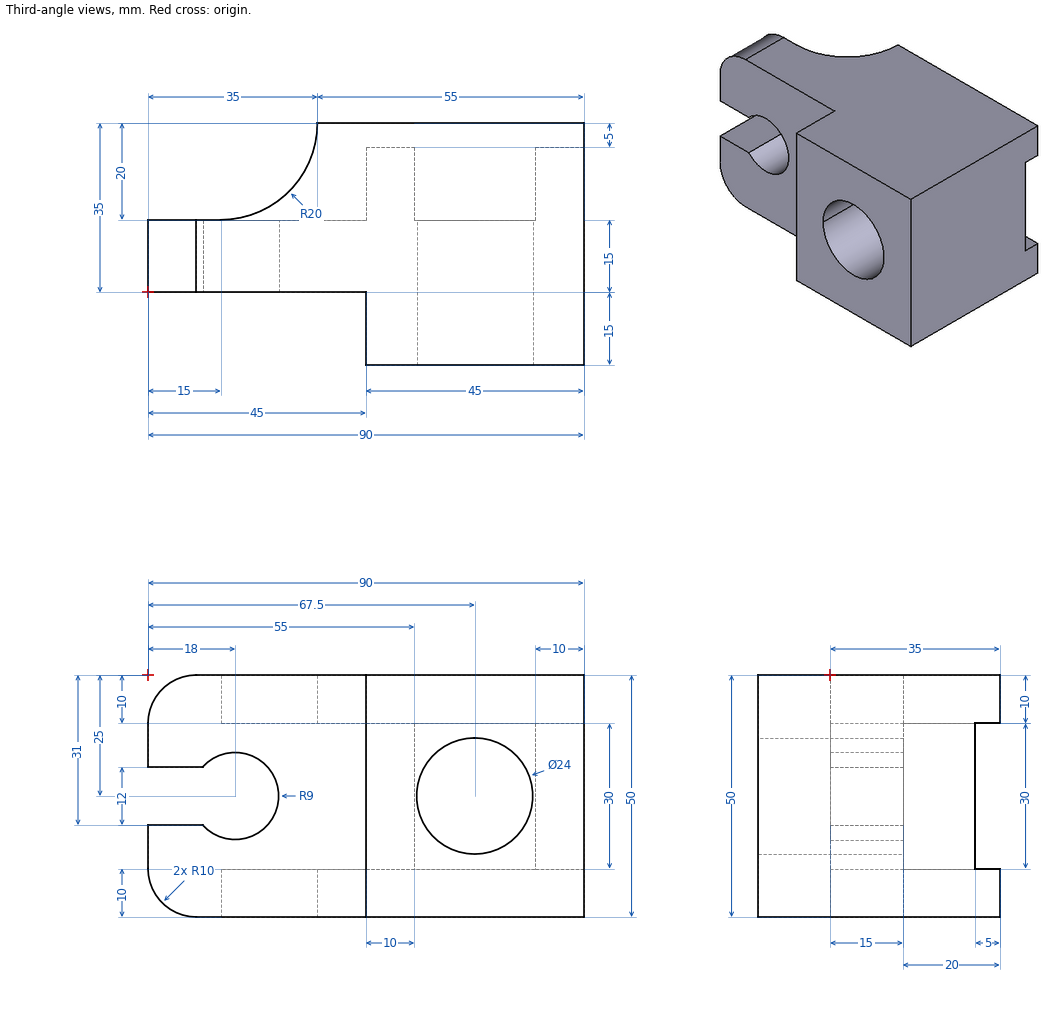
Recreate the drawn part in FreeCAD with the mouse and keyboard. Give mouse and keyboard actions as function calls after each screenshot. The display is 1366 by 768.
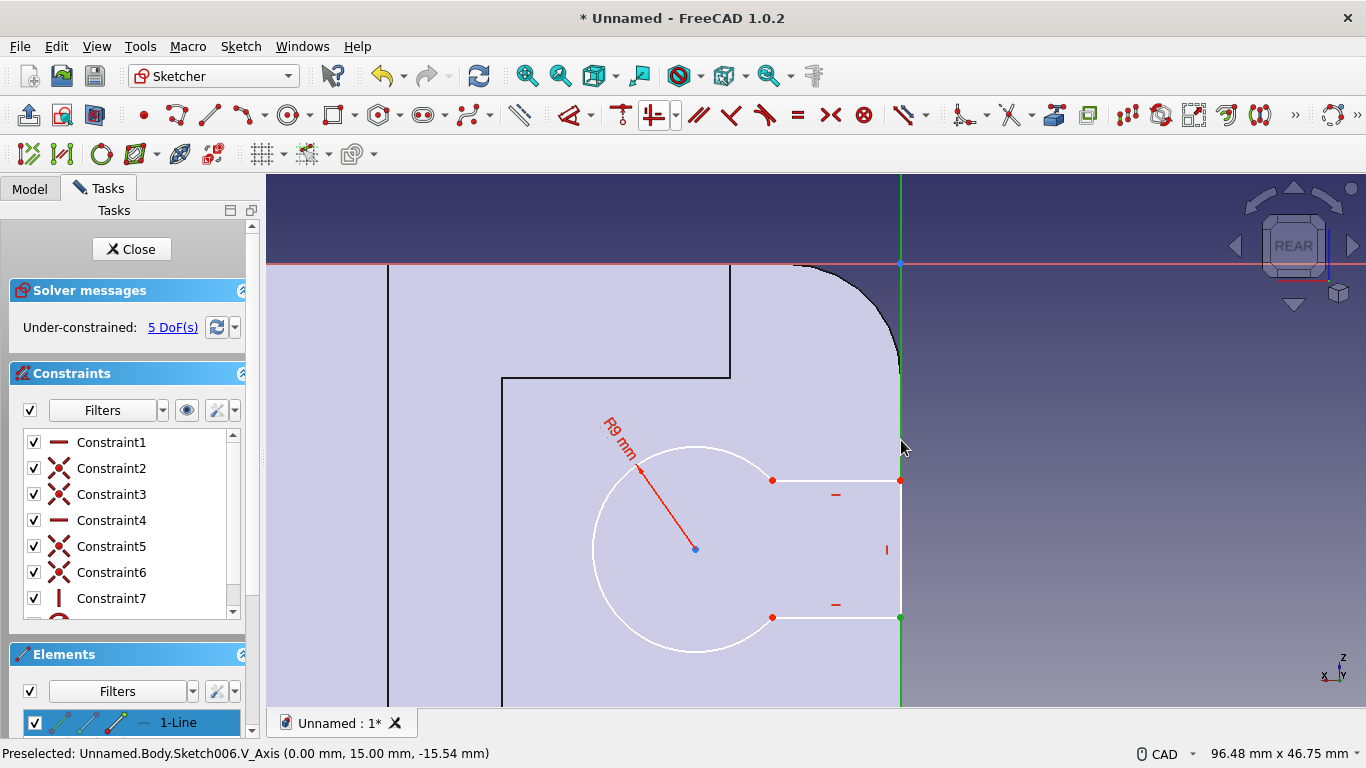
click(621, 116)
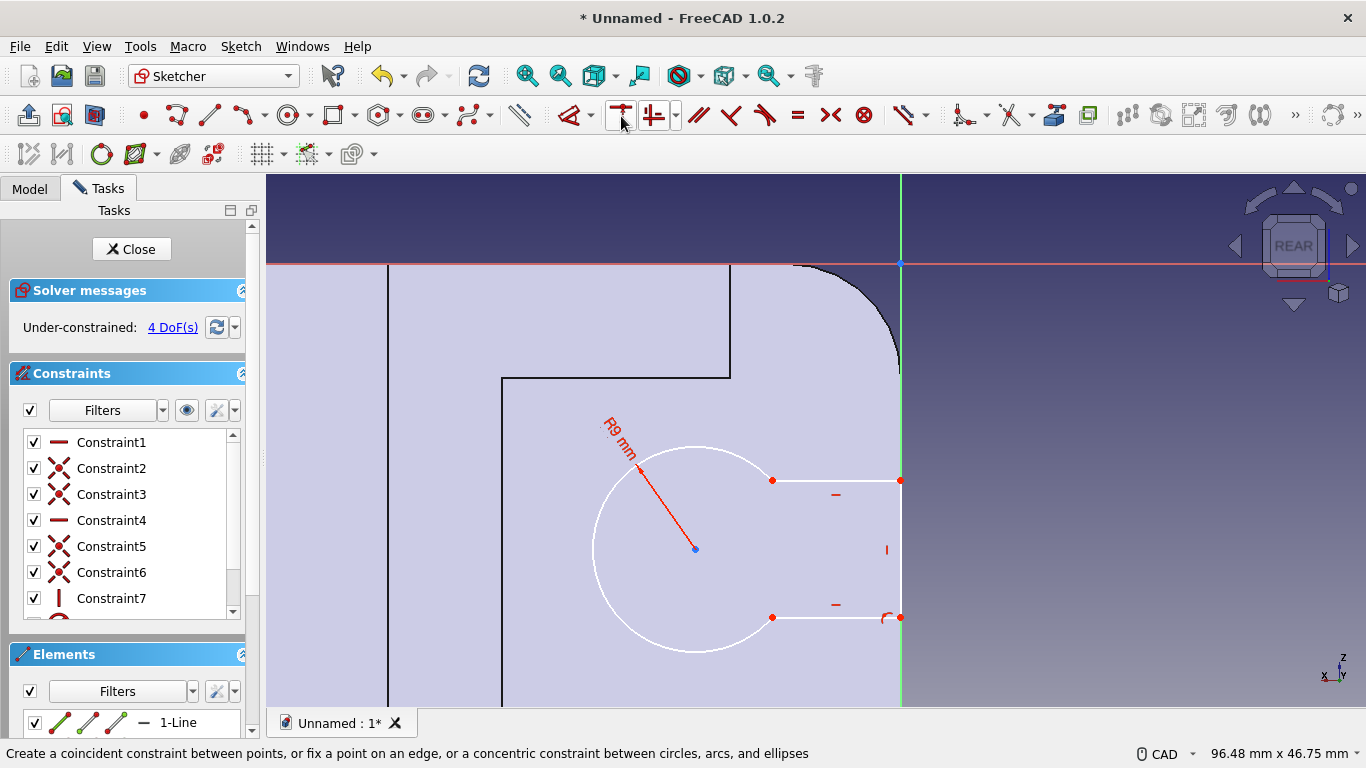
click(568, 116)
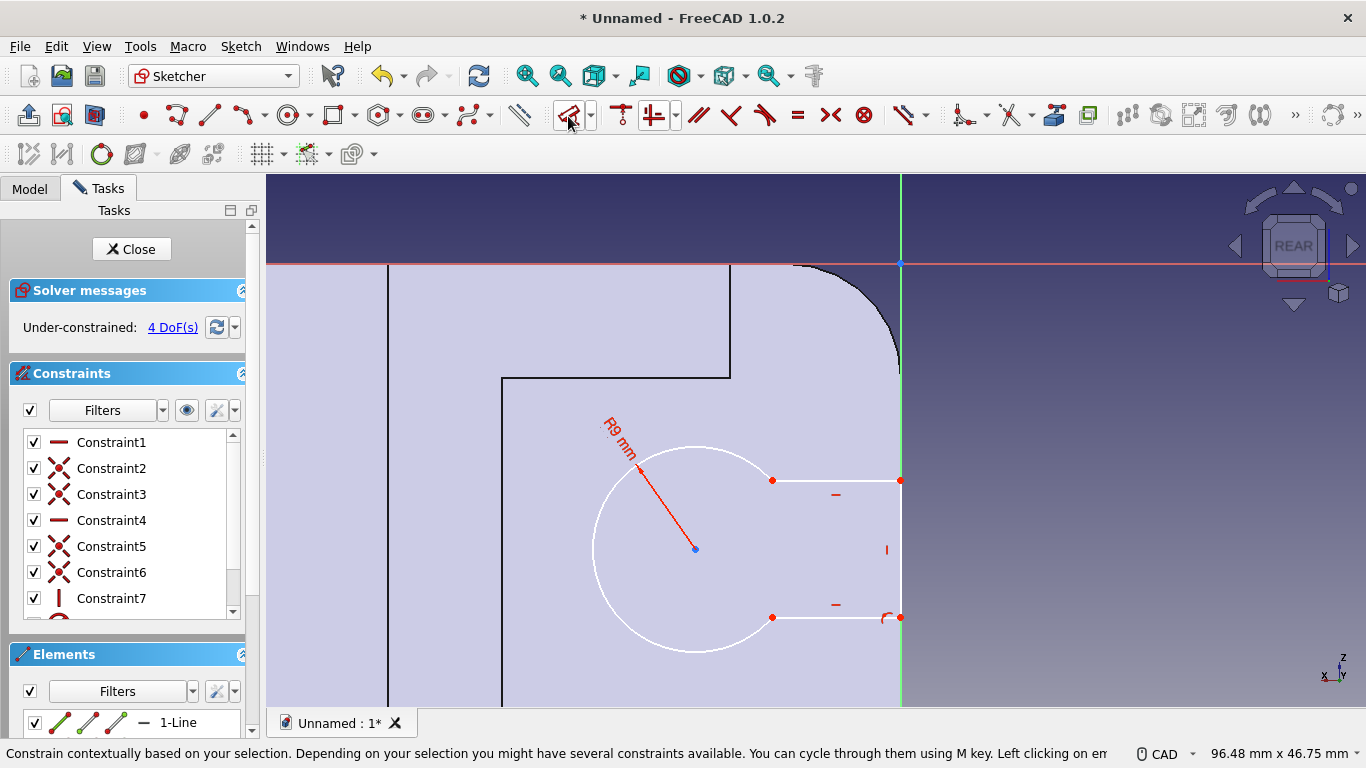
click(901, 577)
click(935, 549)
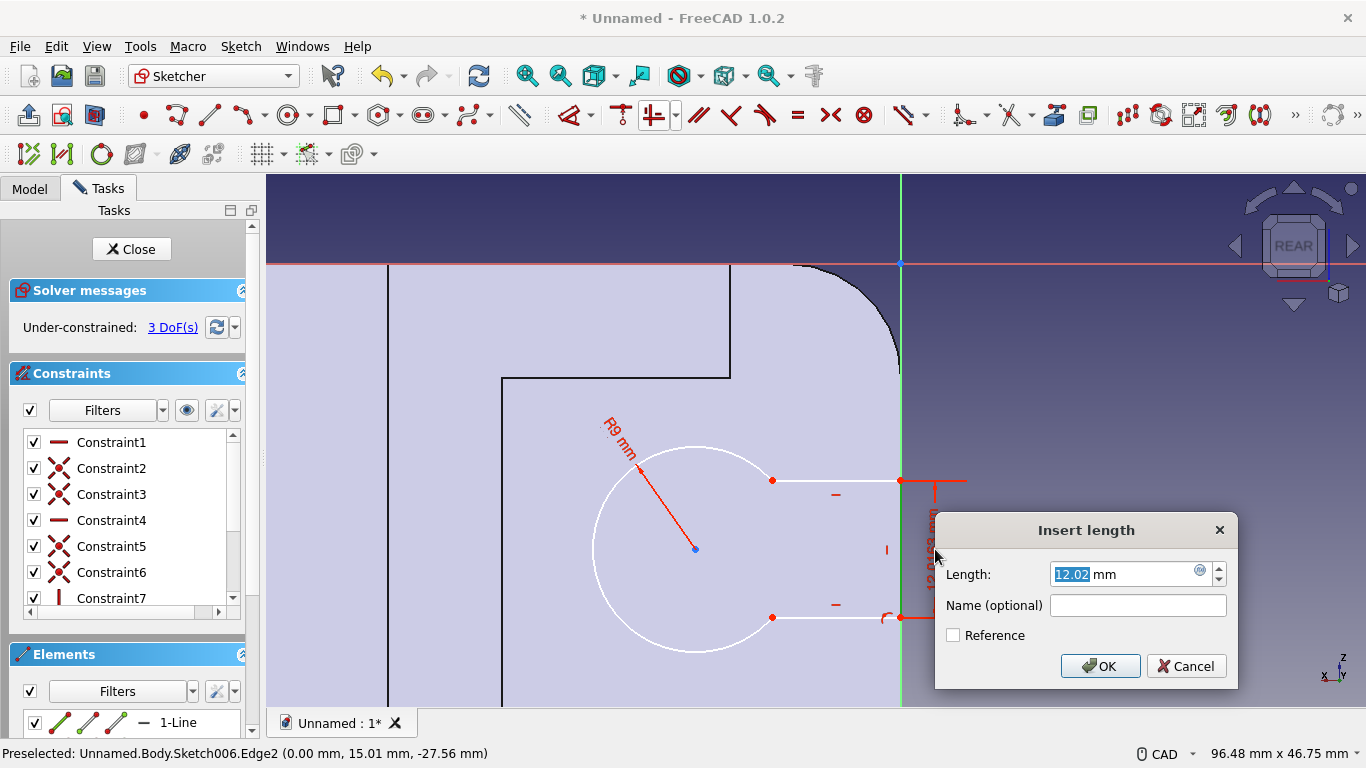
text(12)
key(Return)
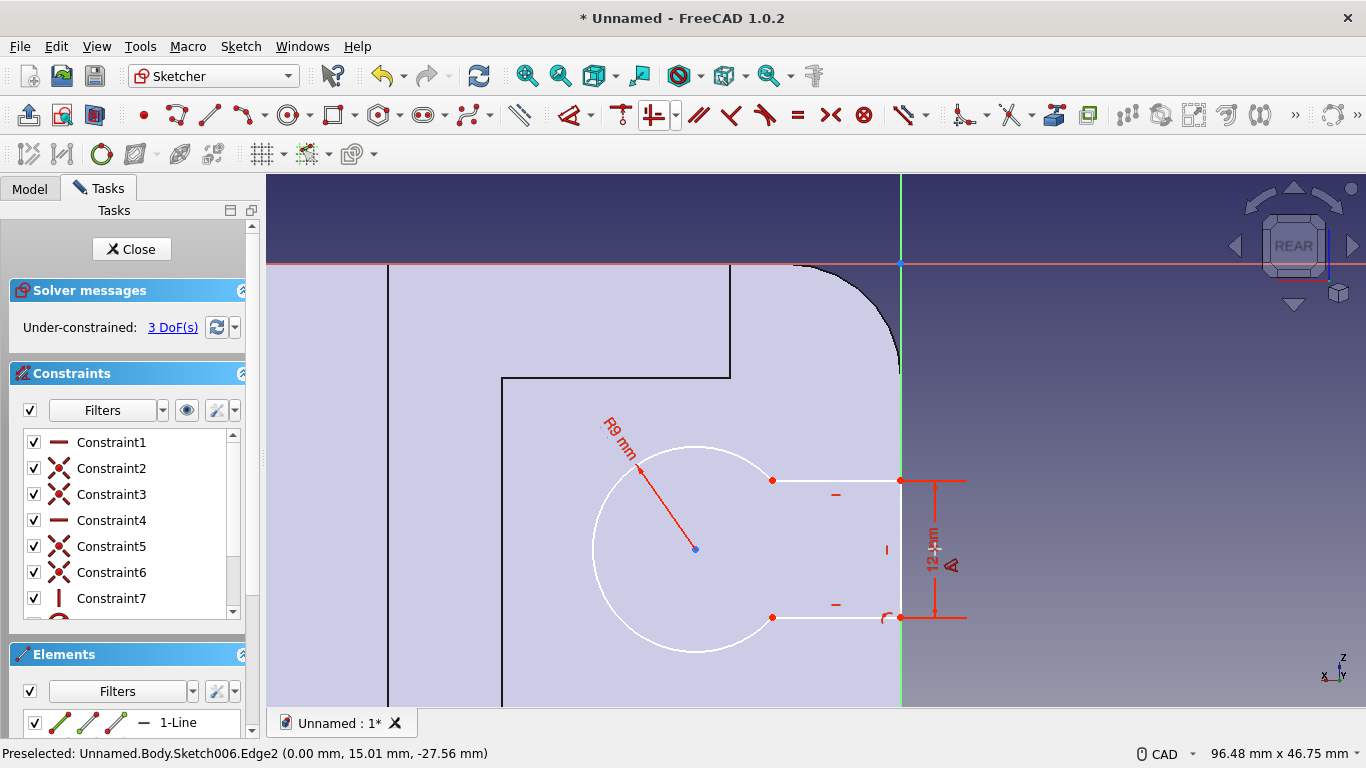
click(772, 618)
click(935, 441)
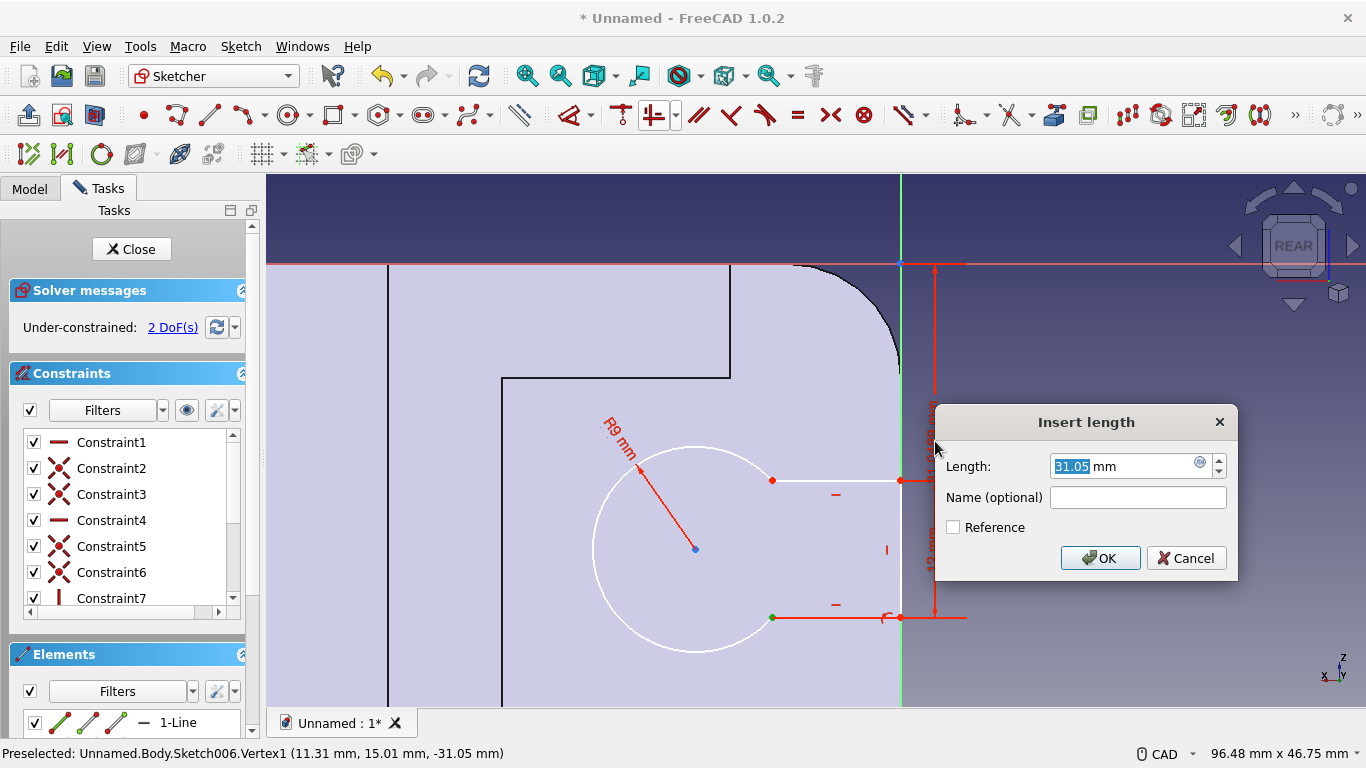
text(31)
key(Return)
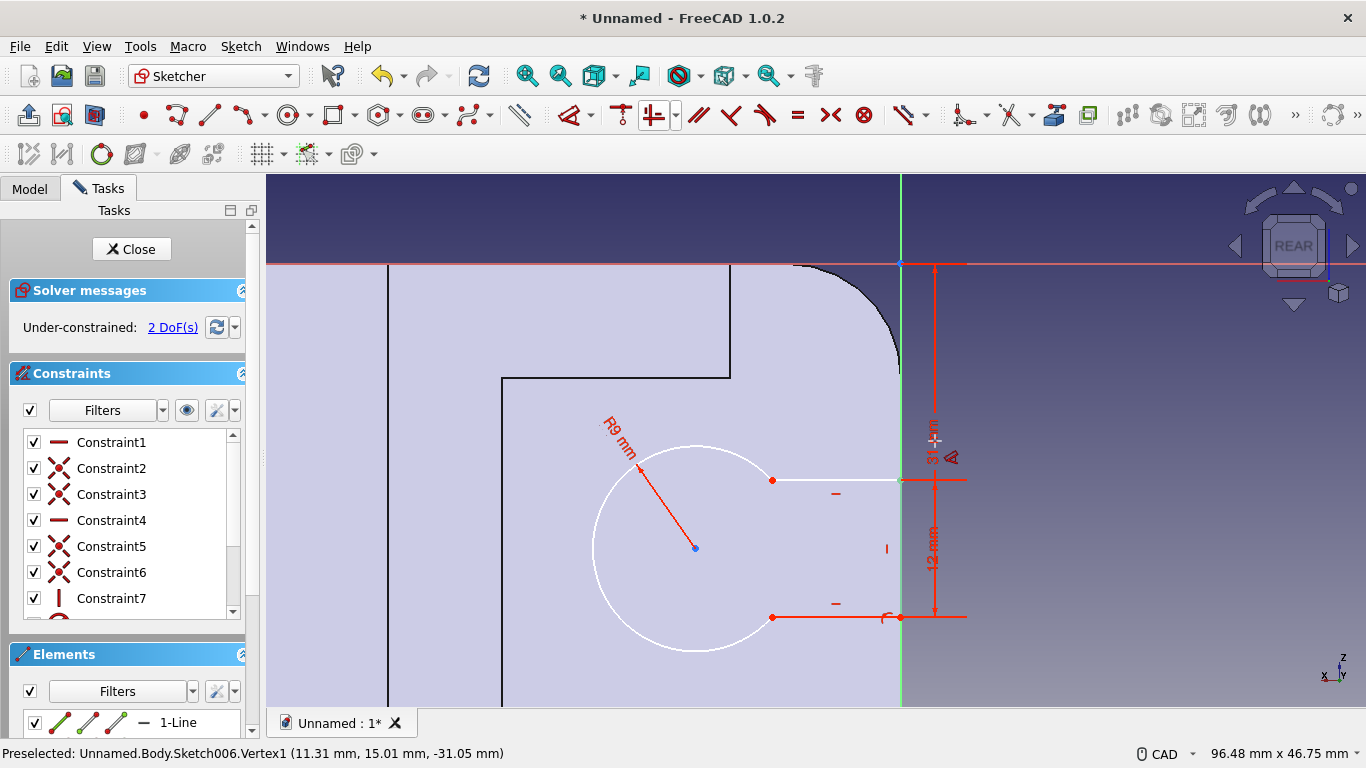
click(696, 549)
click(798, 230)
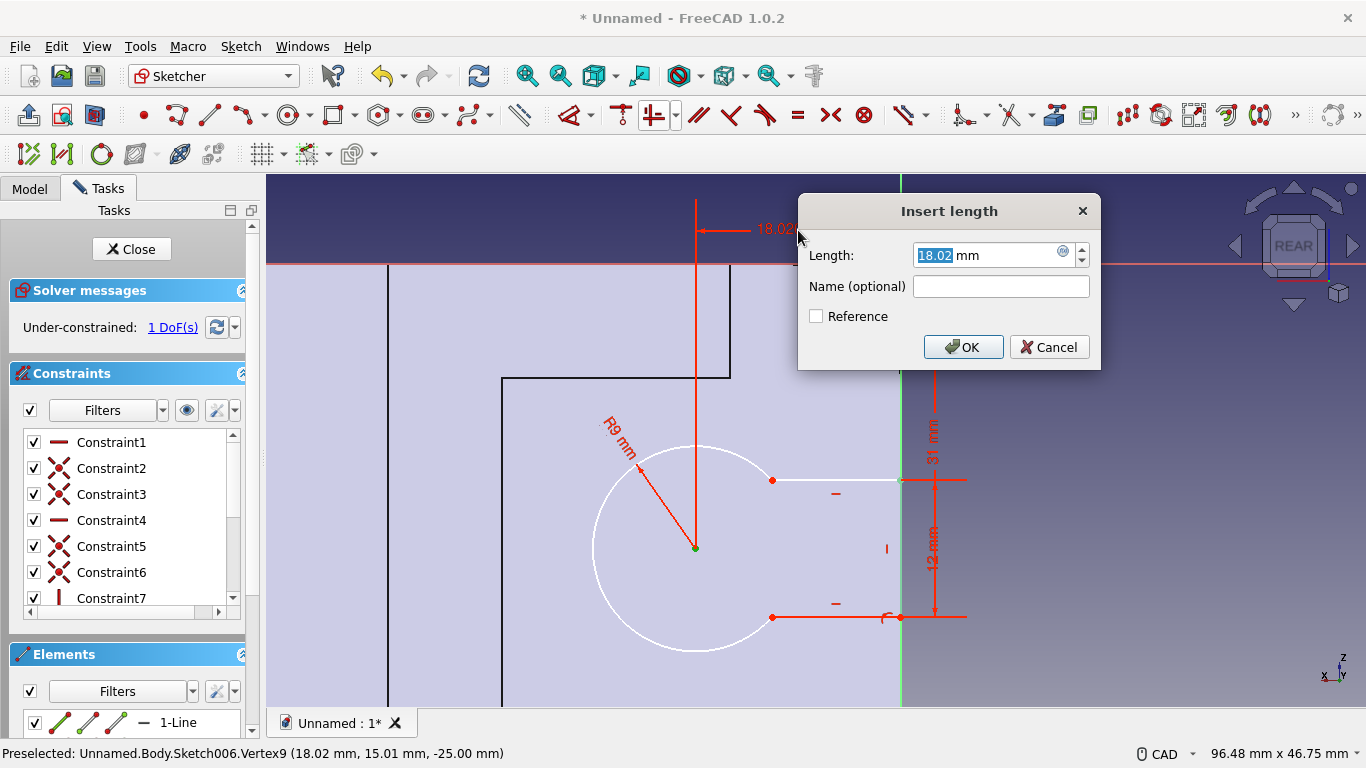
text(18)
key(Return)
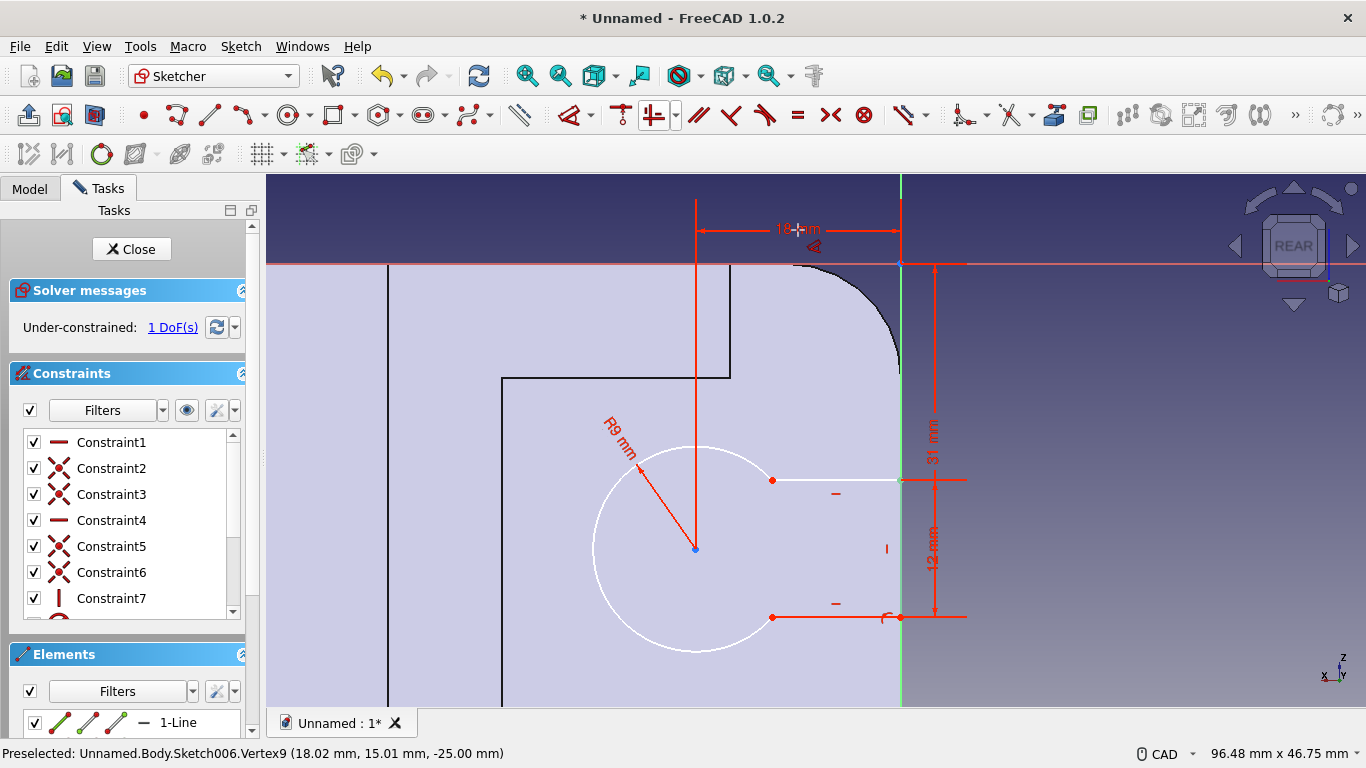
click(696, 549)
click(935, 406)